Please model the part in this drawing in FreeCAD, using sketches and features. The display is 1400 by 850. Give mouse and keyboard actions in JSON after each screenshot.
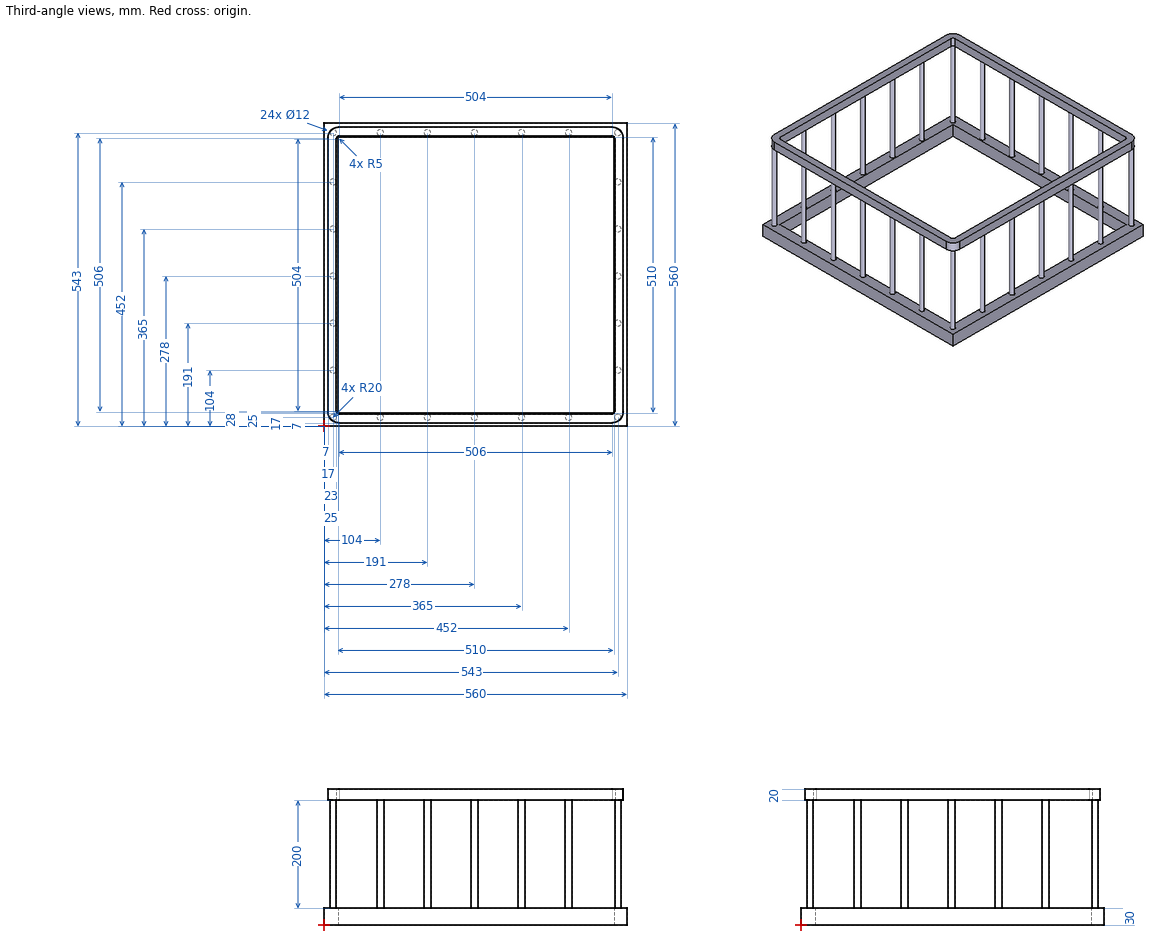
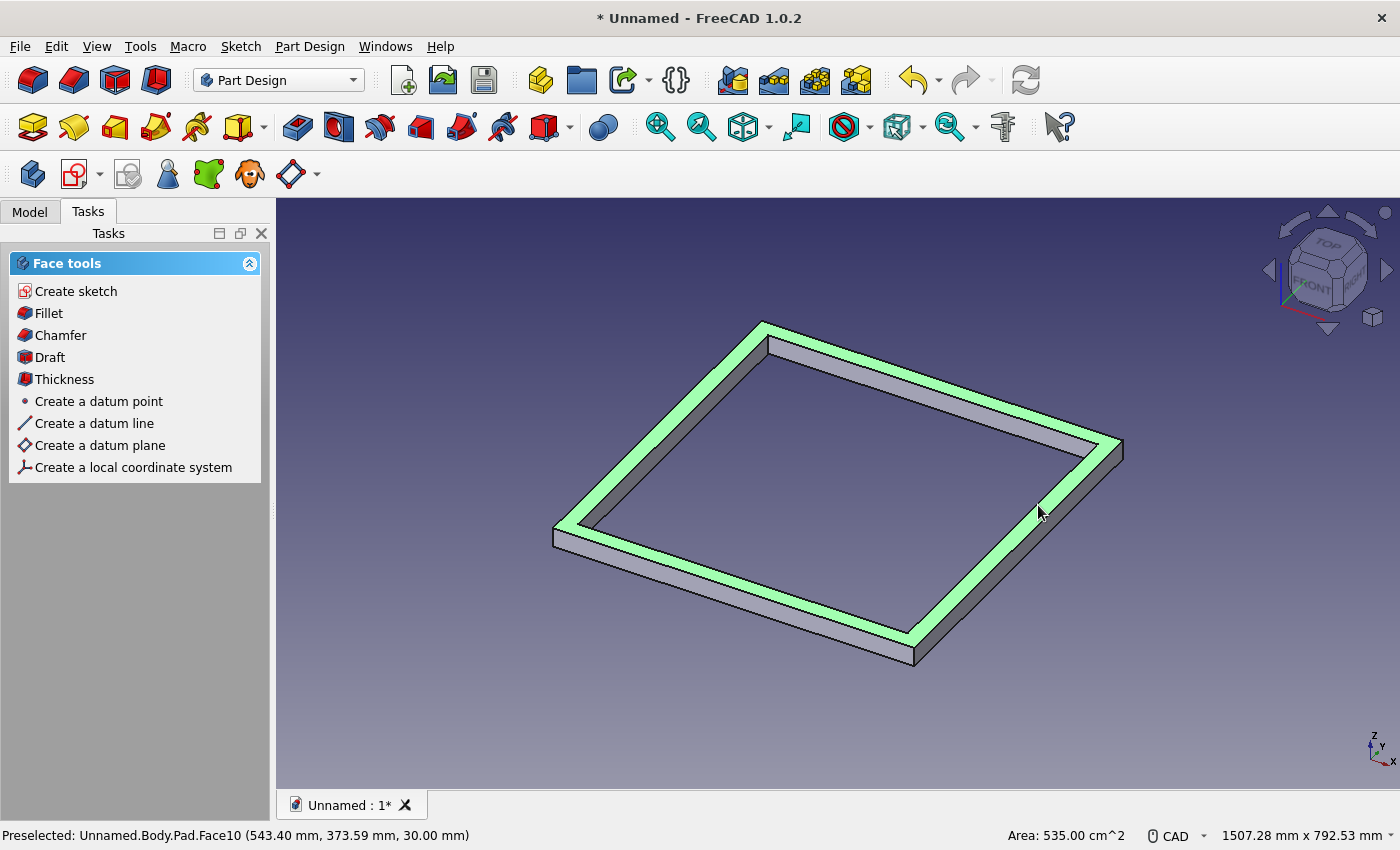
{"action": "left_click", "coordinate": [74, 174]}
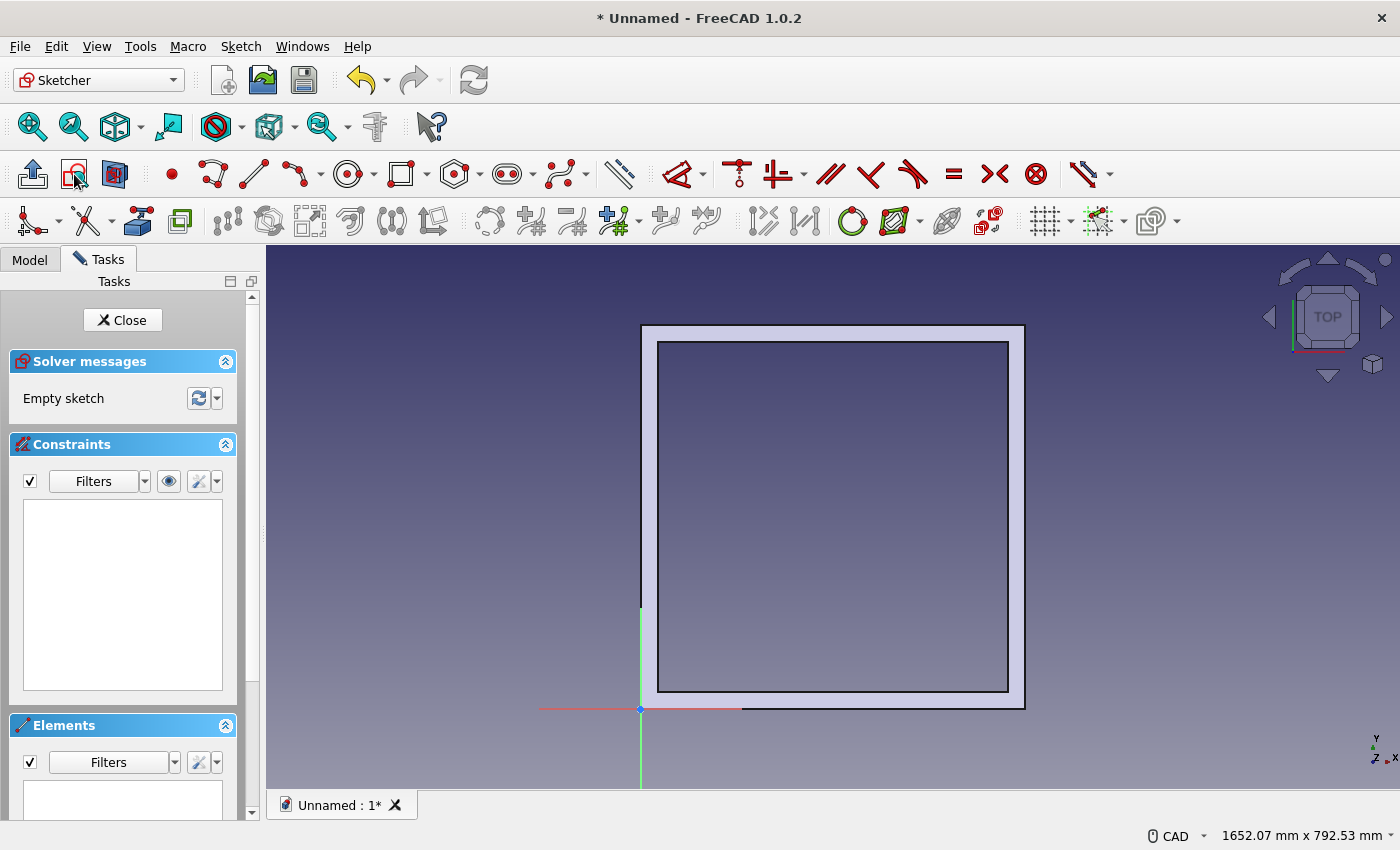
{"action": "left_click", "coordinate": [348, 174]}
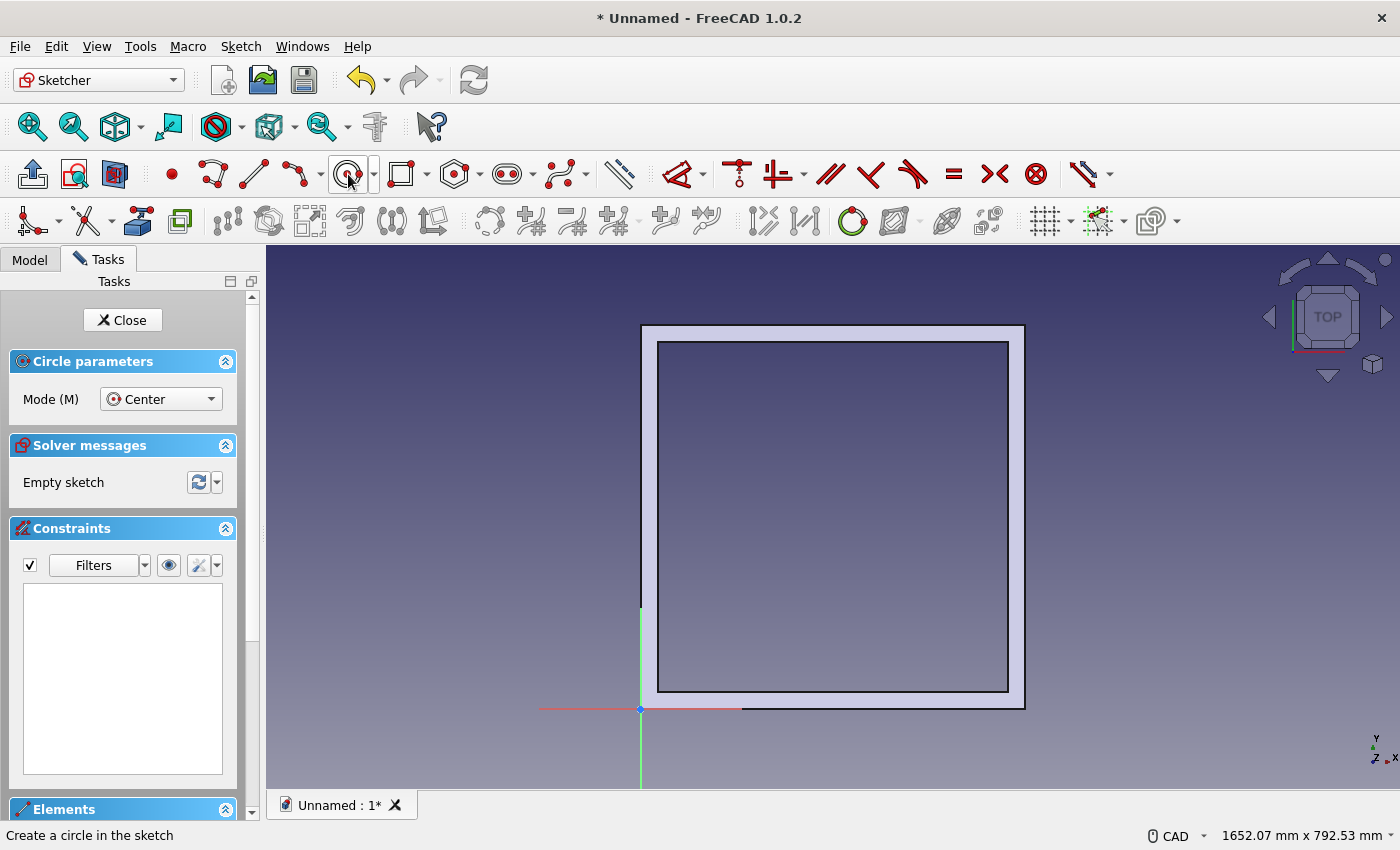
{"action": "scroll", "coordinate": [652, 336], "scroll_direction": "up", "scroll_amount": 9}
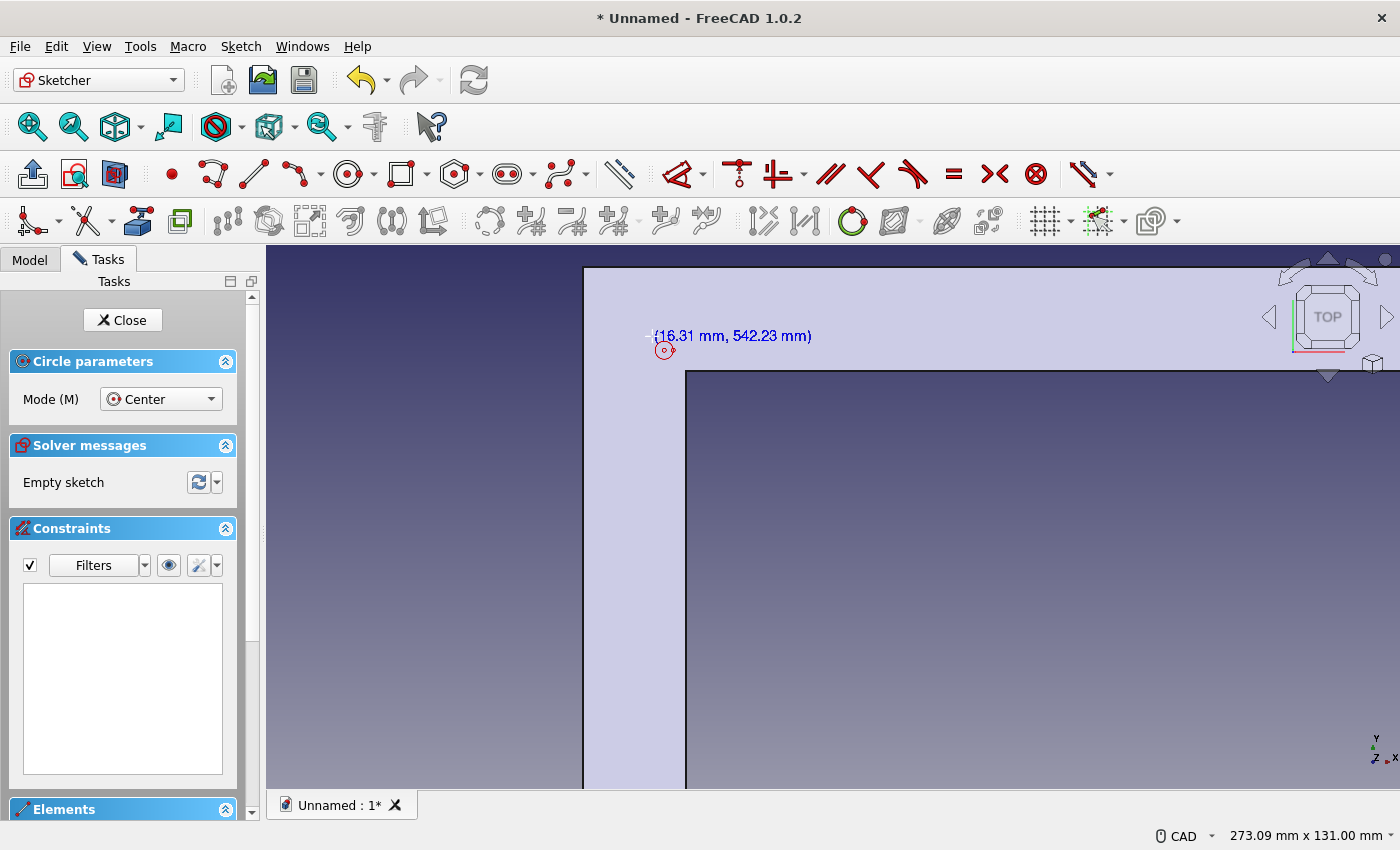
{"action": "scroll", "coordinate": [575, 332], "scroll_direction": "down", "scroll_amount": 9}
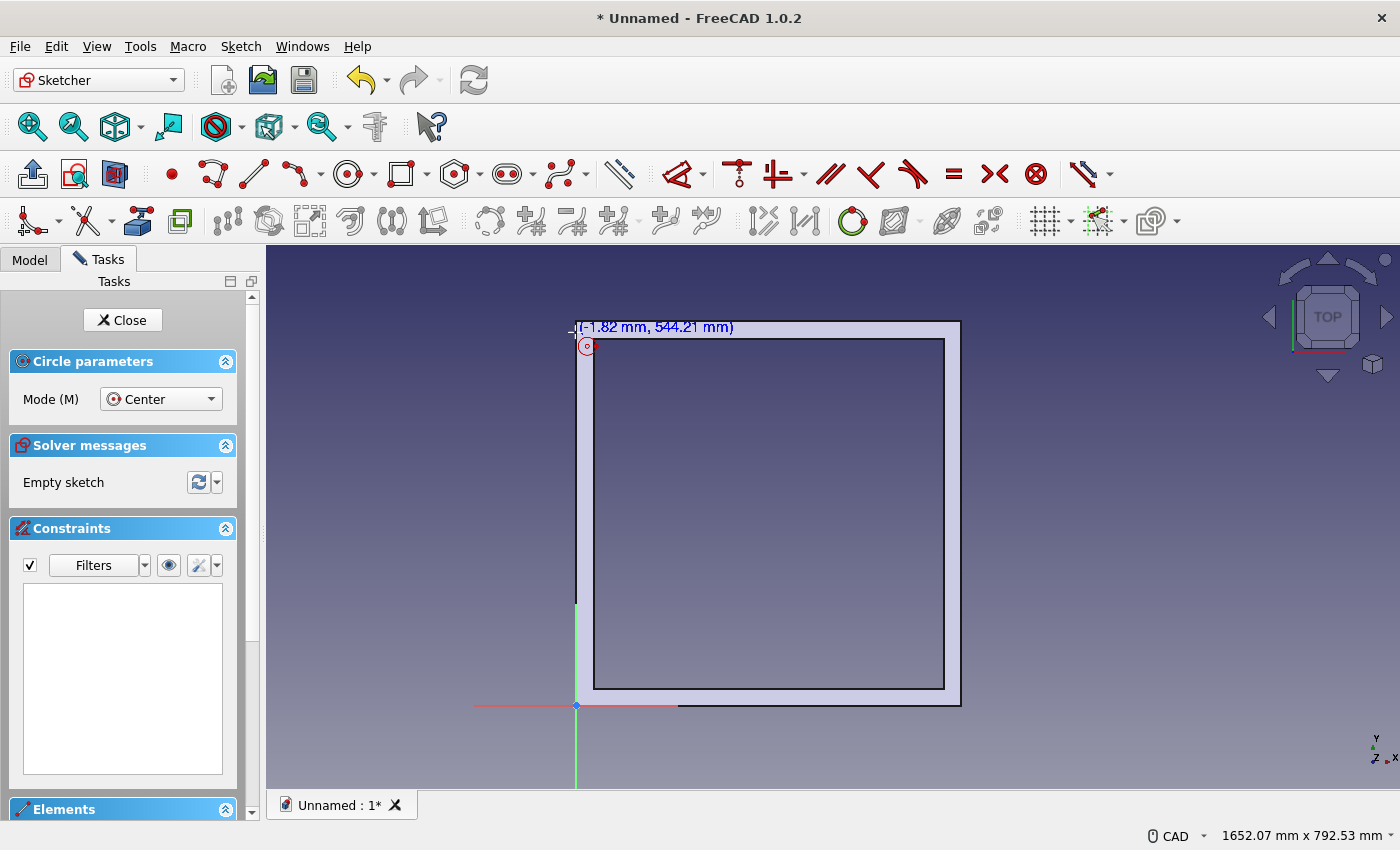
{"action": "scroll", "coordinate": [588, 333], "scroll_direction": "up", "scroll_amount": 2}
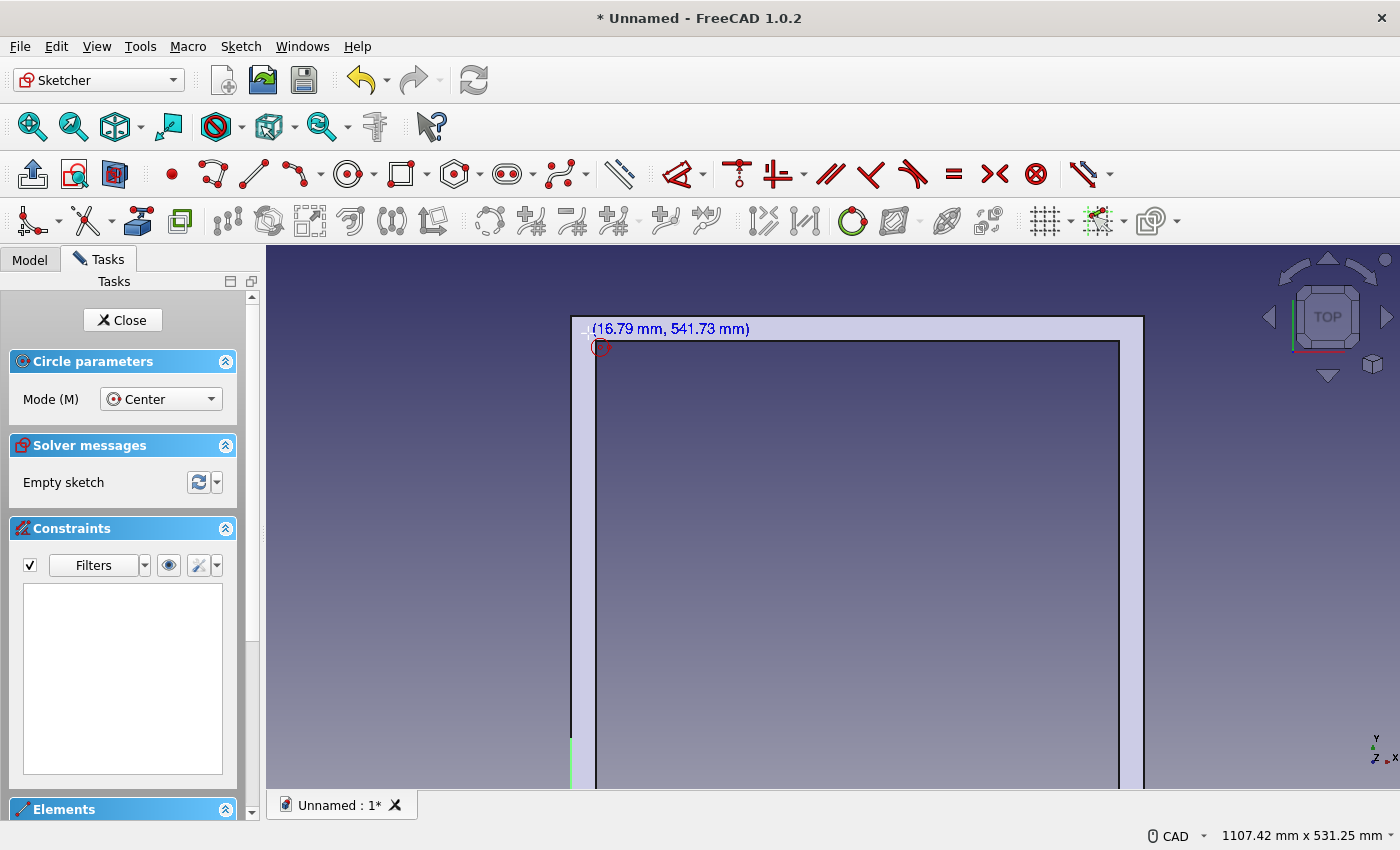
{"action": "left_click", "coordinate": [588, 333]}
{"action": "mouse_move", "coordinate": [592, 329]}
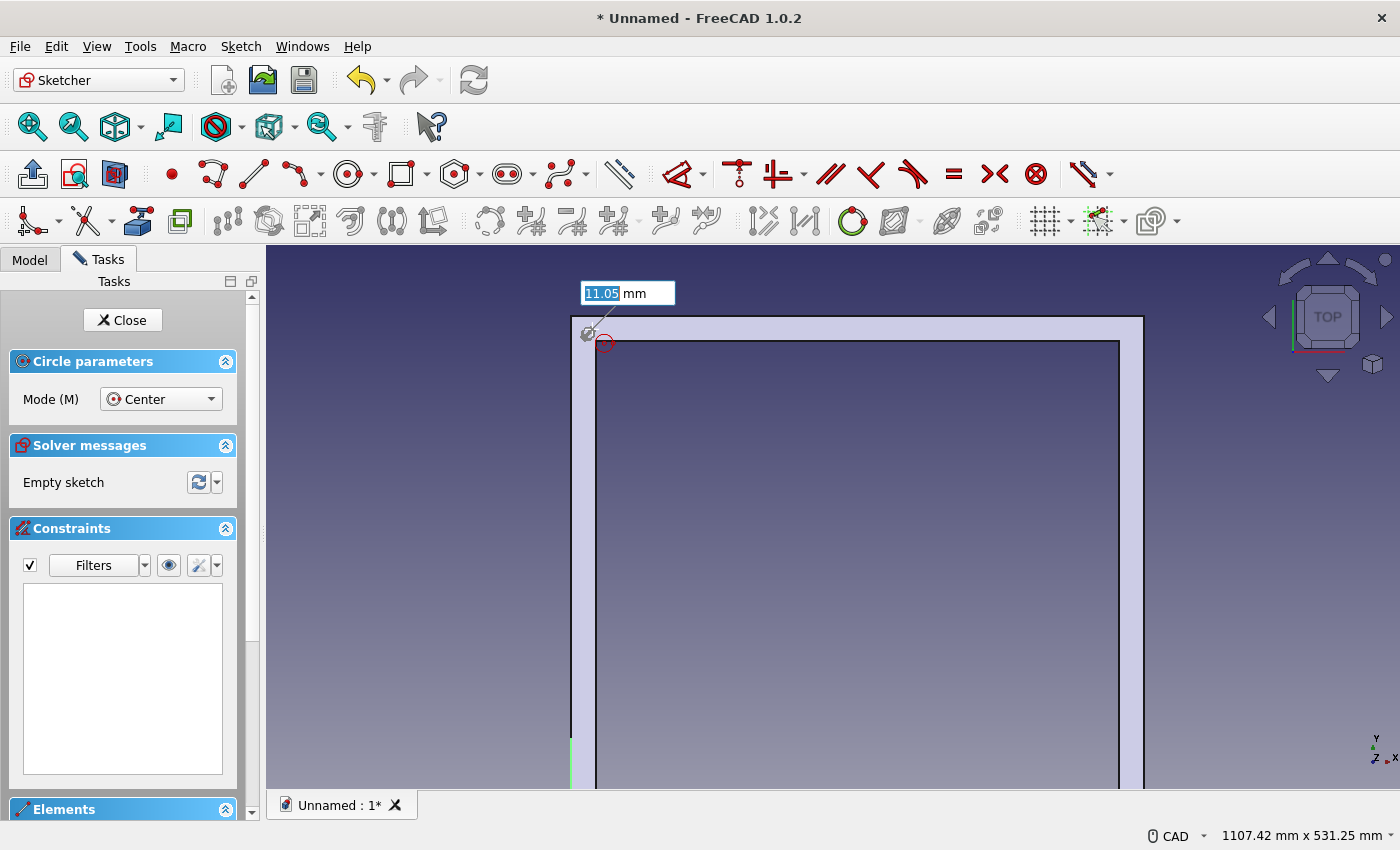
{"action": "type", "text": "12"}
{"action": "key", "text": "Return"}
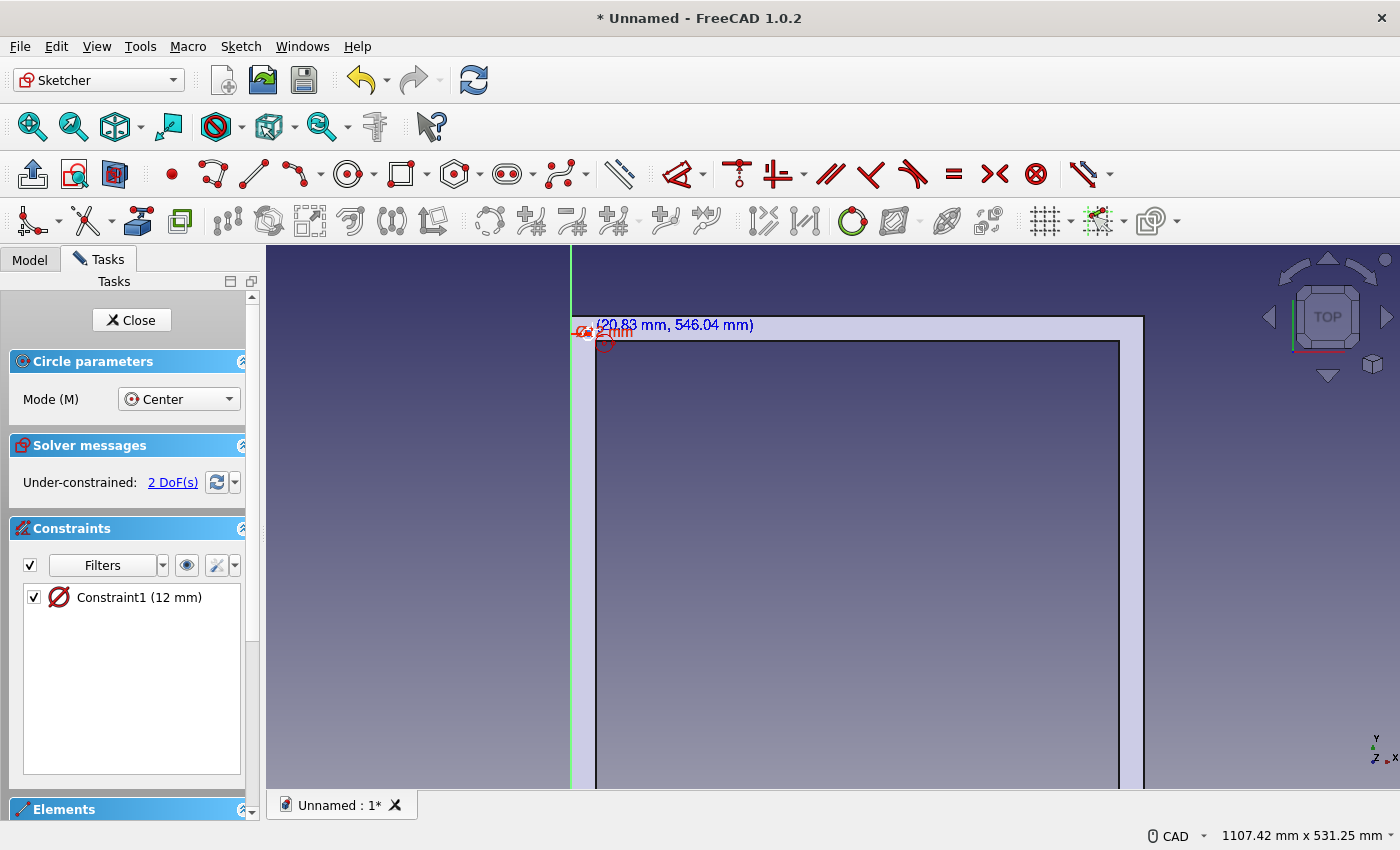
{"action": "scroll", "coordinate": [587, 332], "scroll_direction": "down", "scroll_amount": 2}